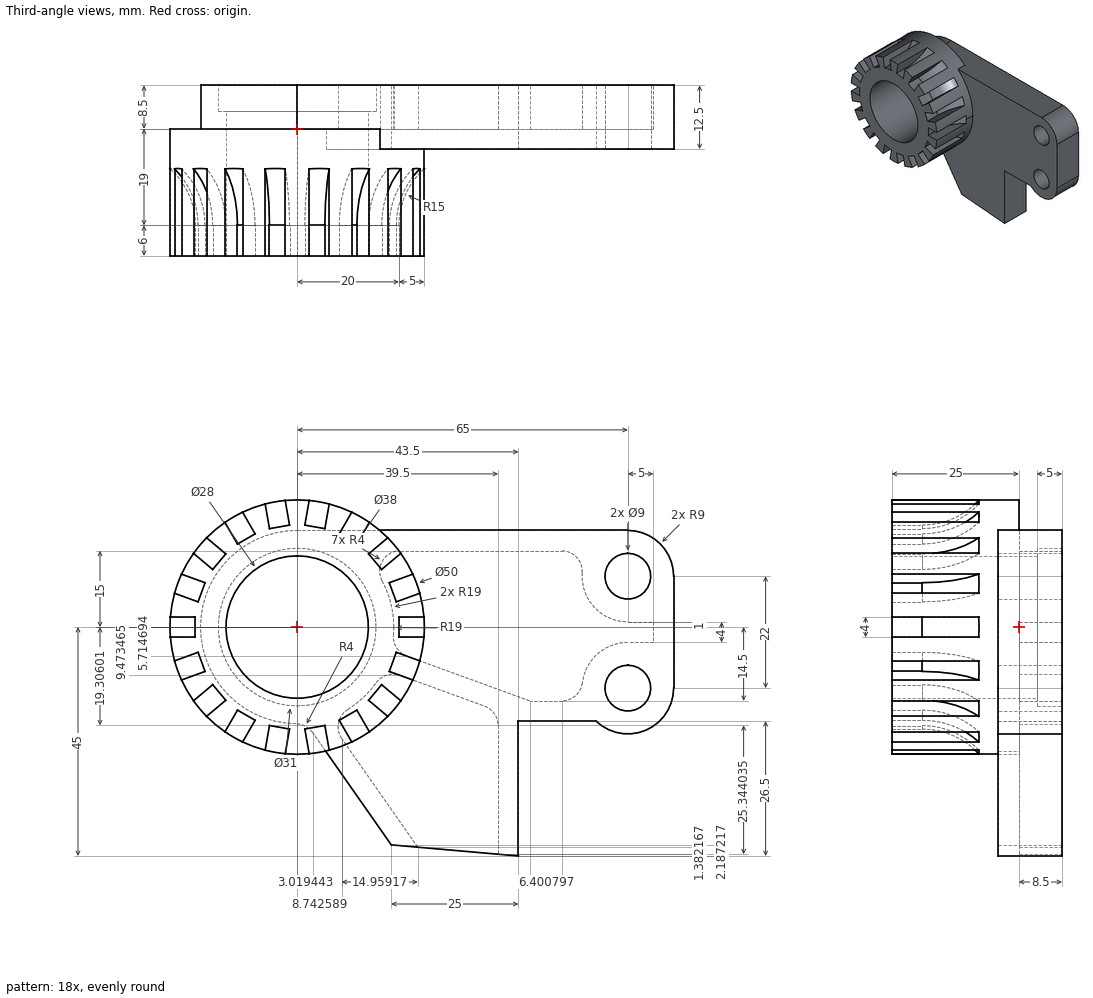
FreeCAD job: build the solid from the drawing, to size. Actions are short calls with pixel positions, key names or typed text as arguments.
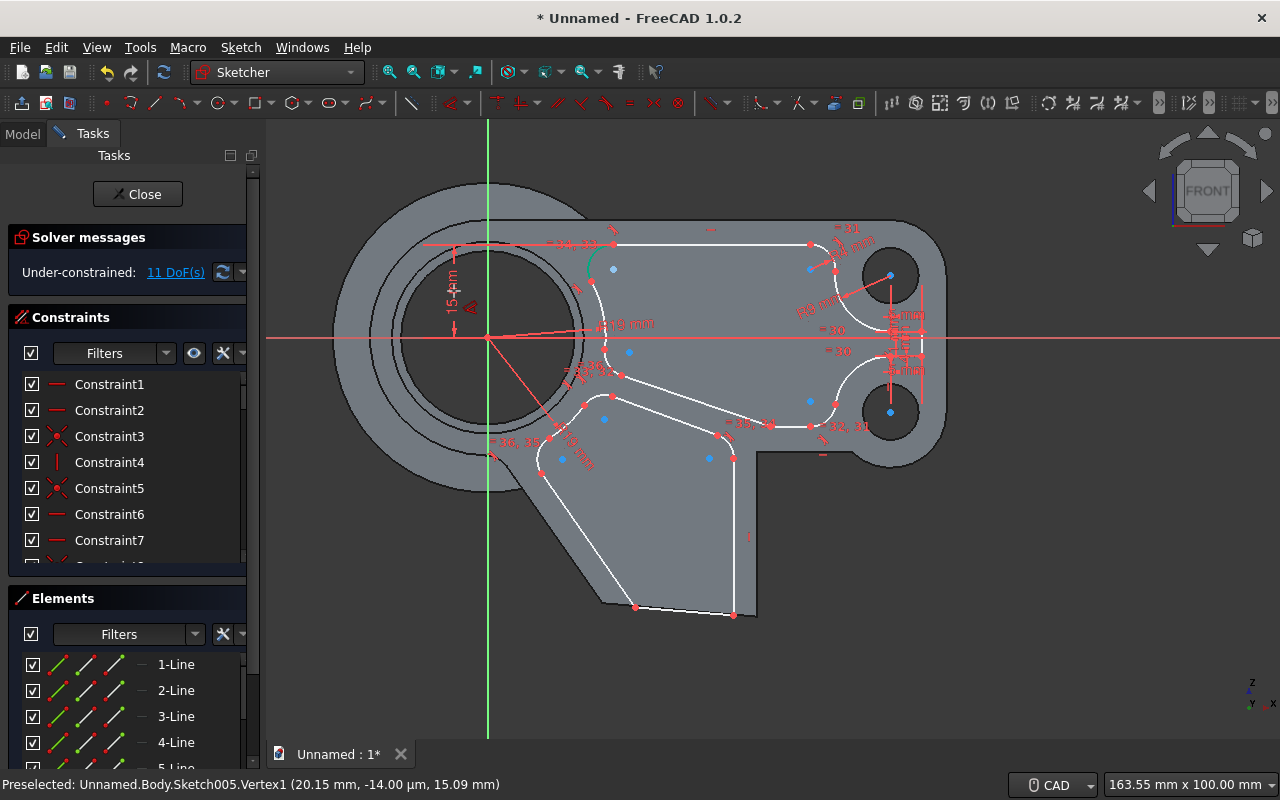
click(891, 332)
click(689, 298)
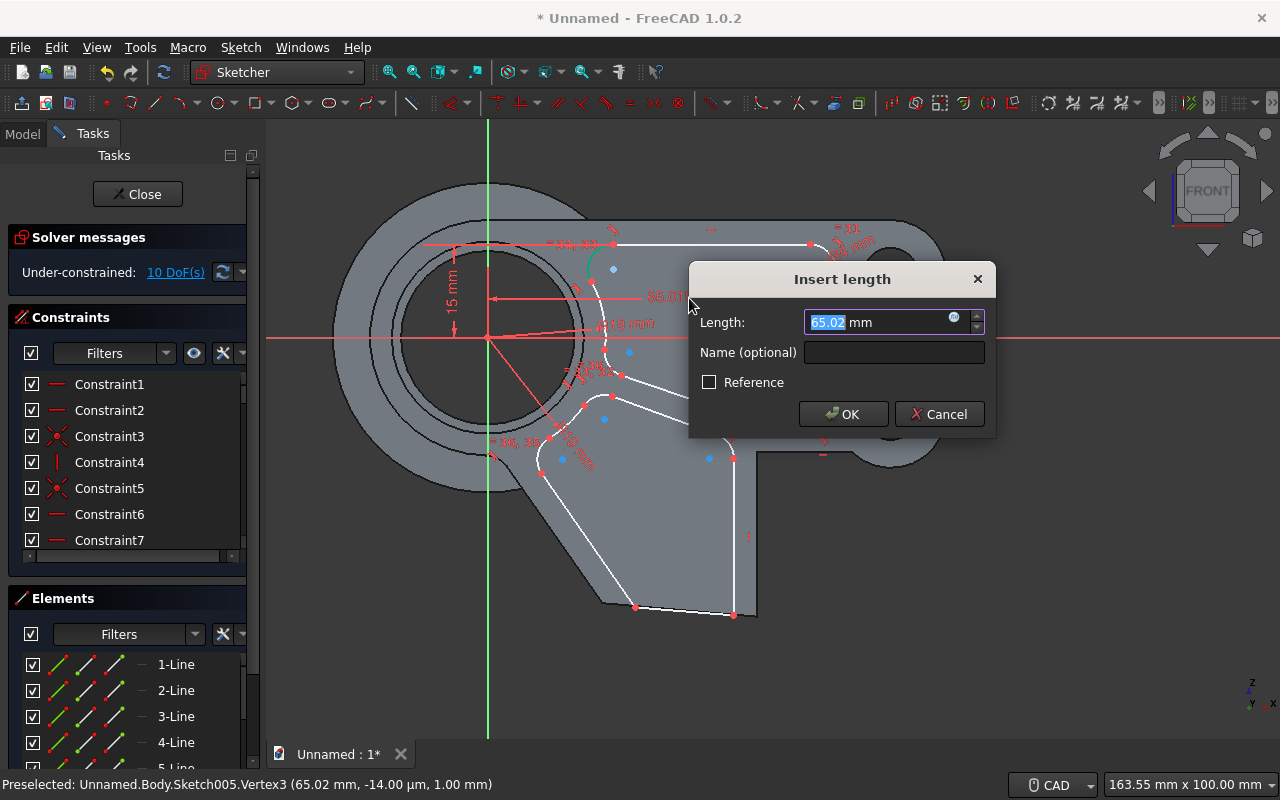
text(65)
key(Return)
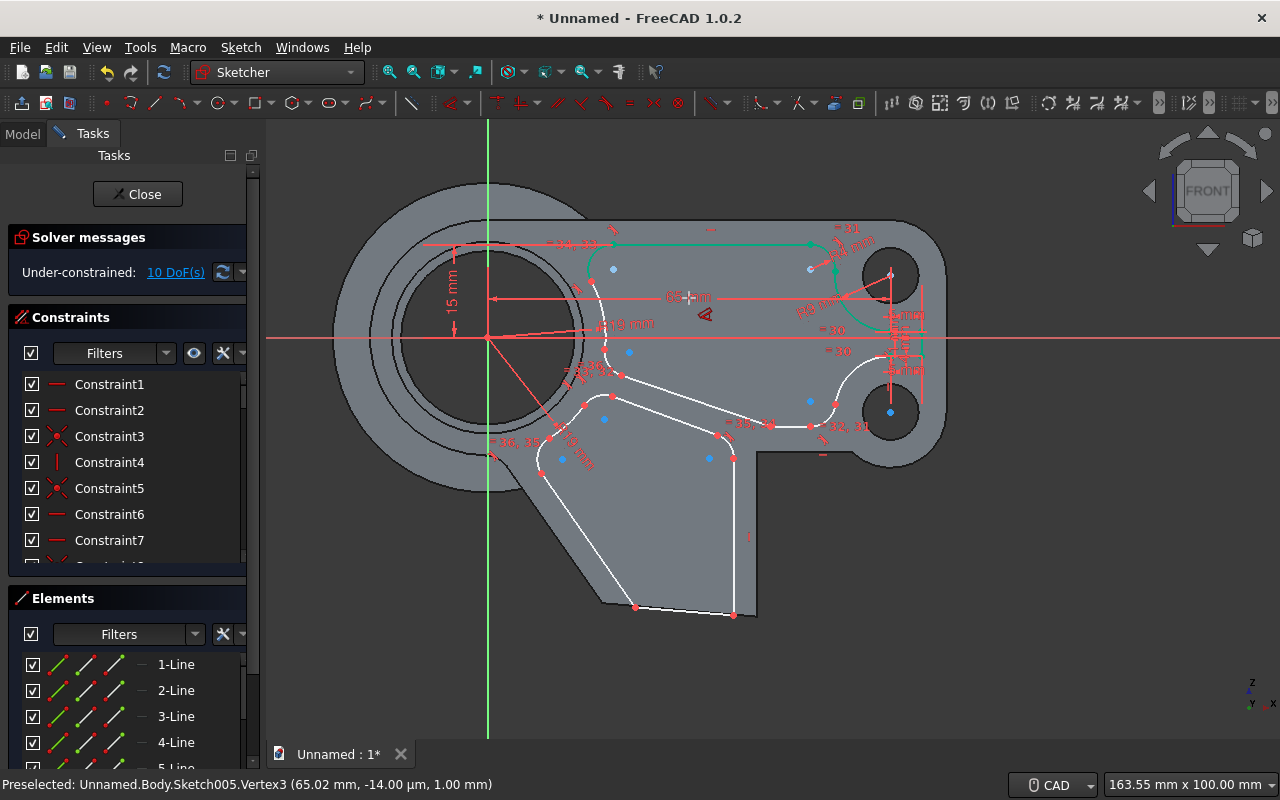
click(811, 427)
click(454, 382)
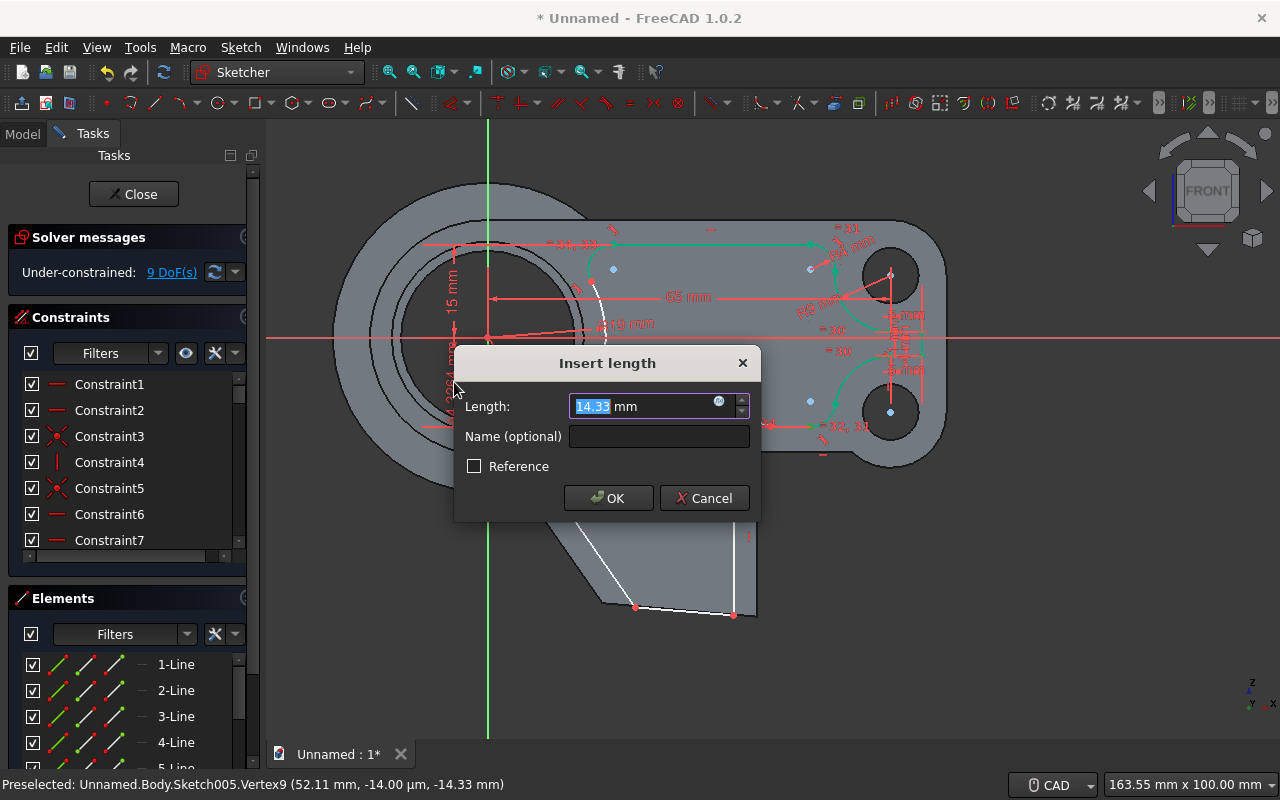
text(14.5)
key(Return)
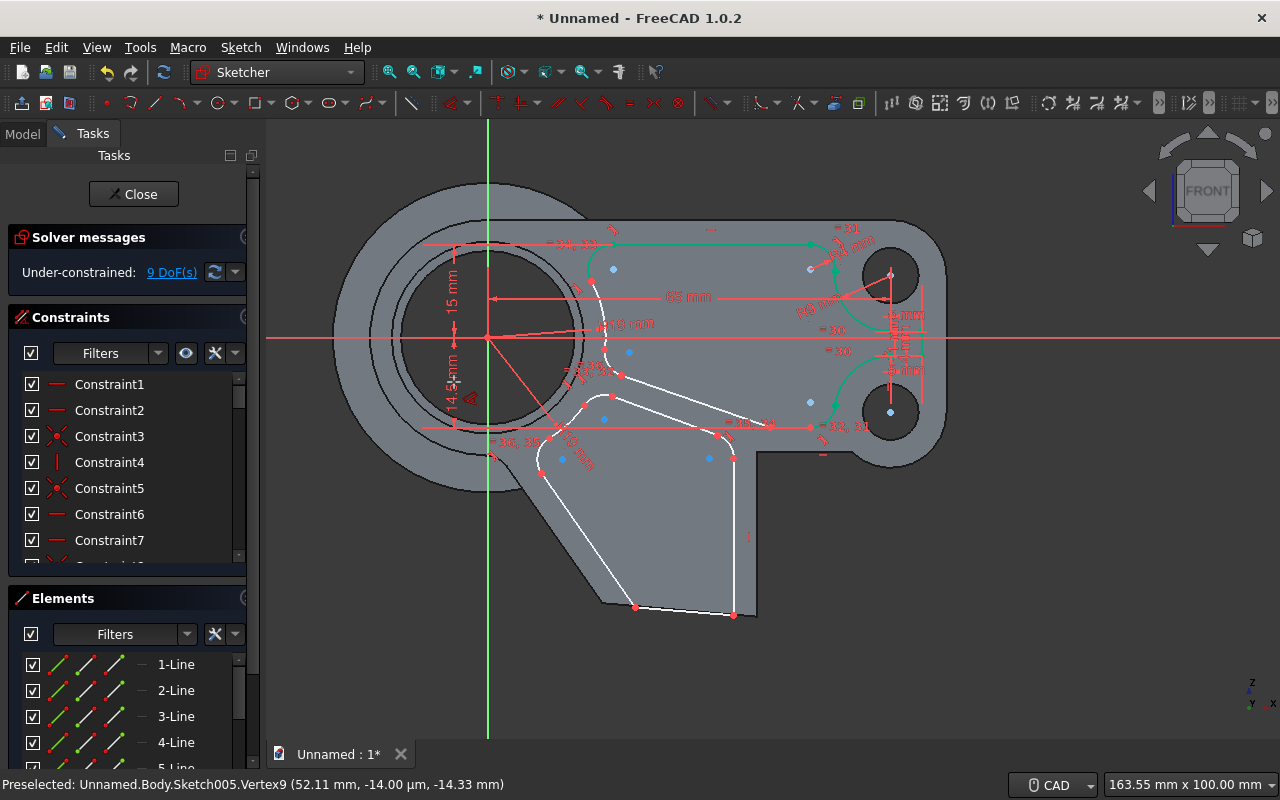
click(734, 458)
click(554, 304)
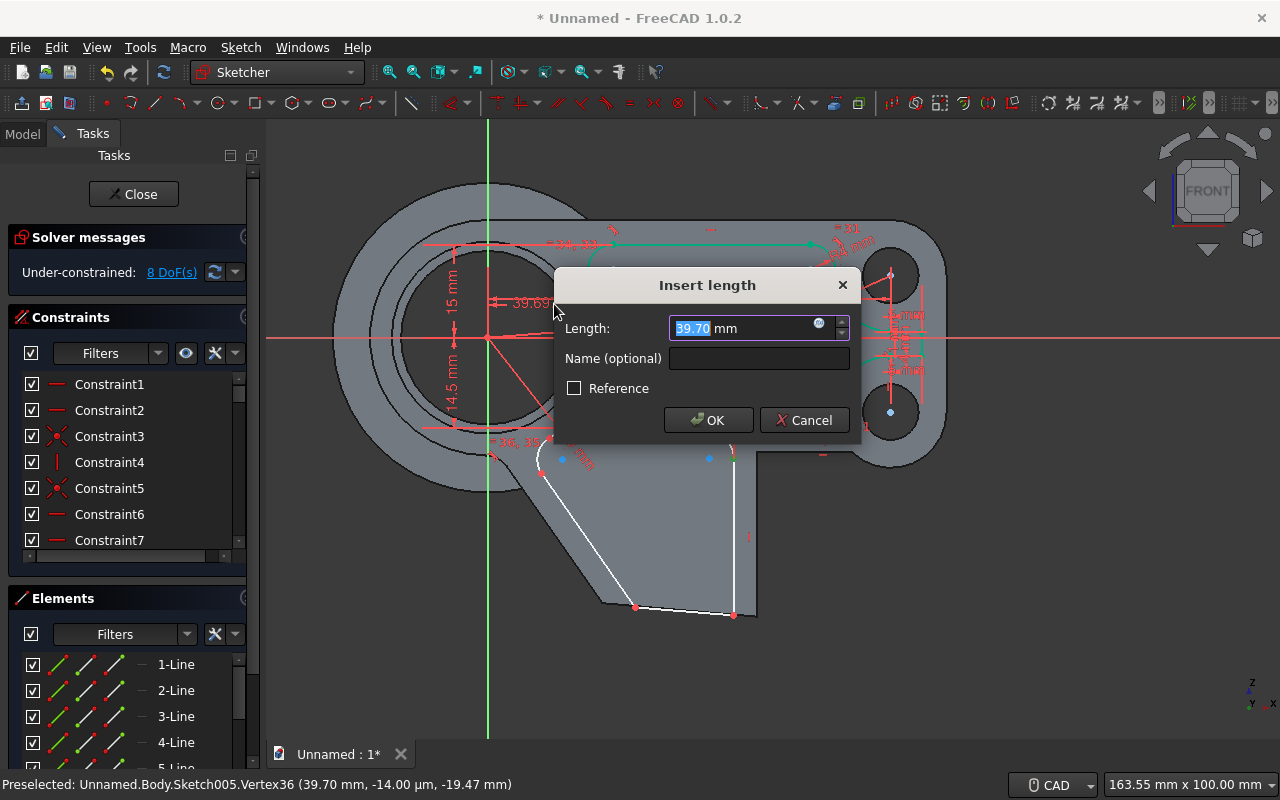
text(39.5)
key(Return)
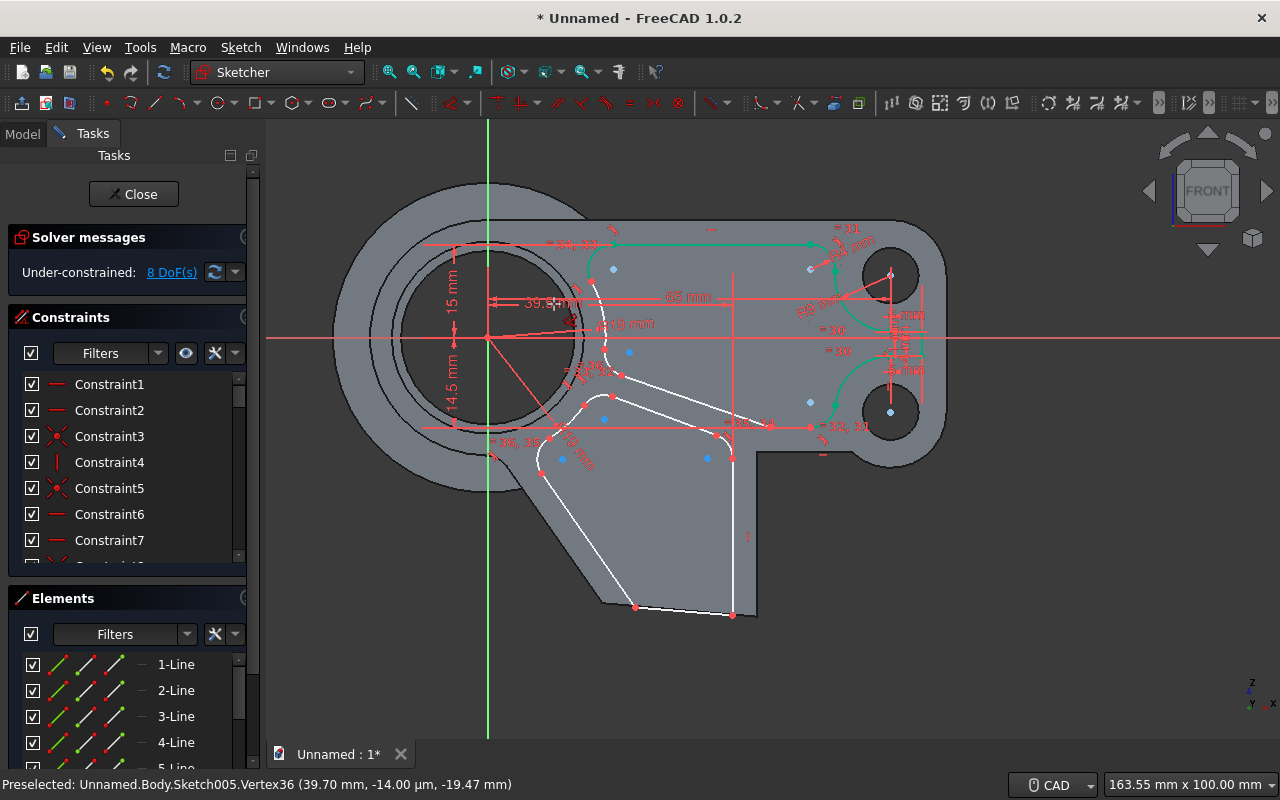
click(799, 428)
click(791, 394)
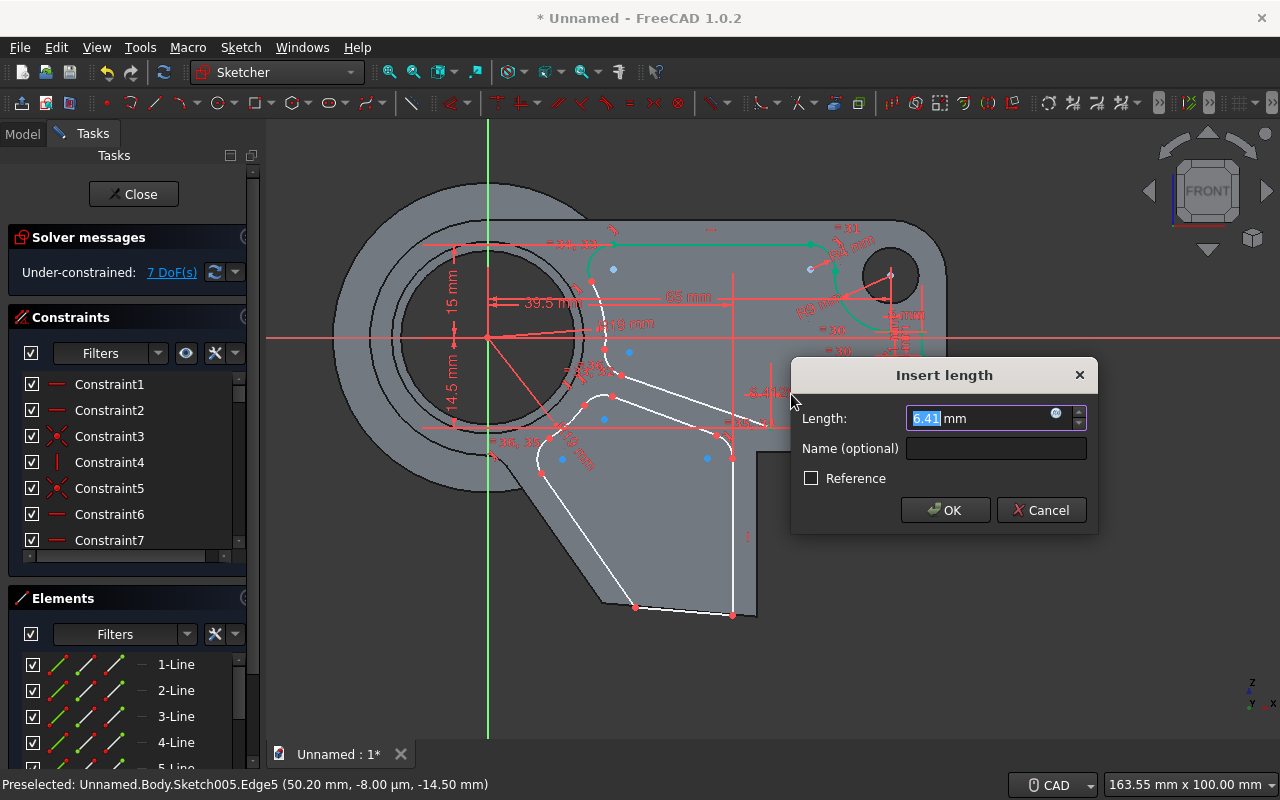
text(6.400797)
key(Return)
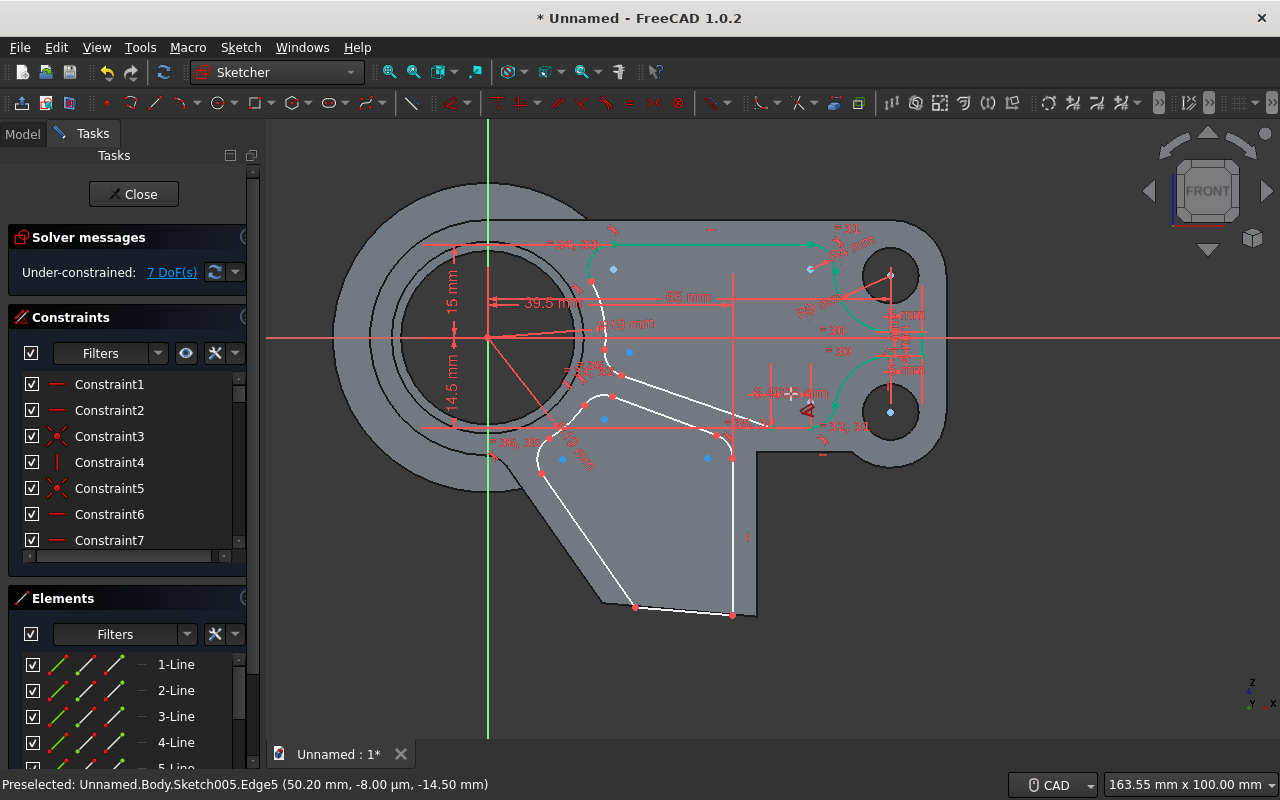
click(733, 506)
click(767, 537)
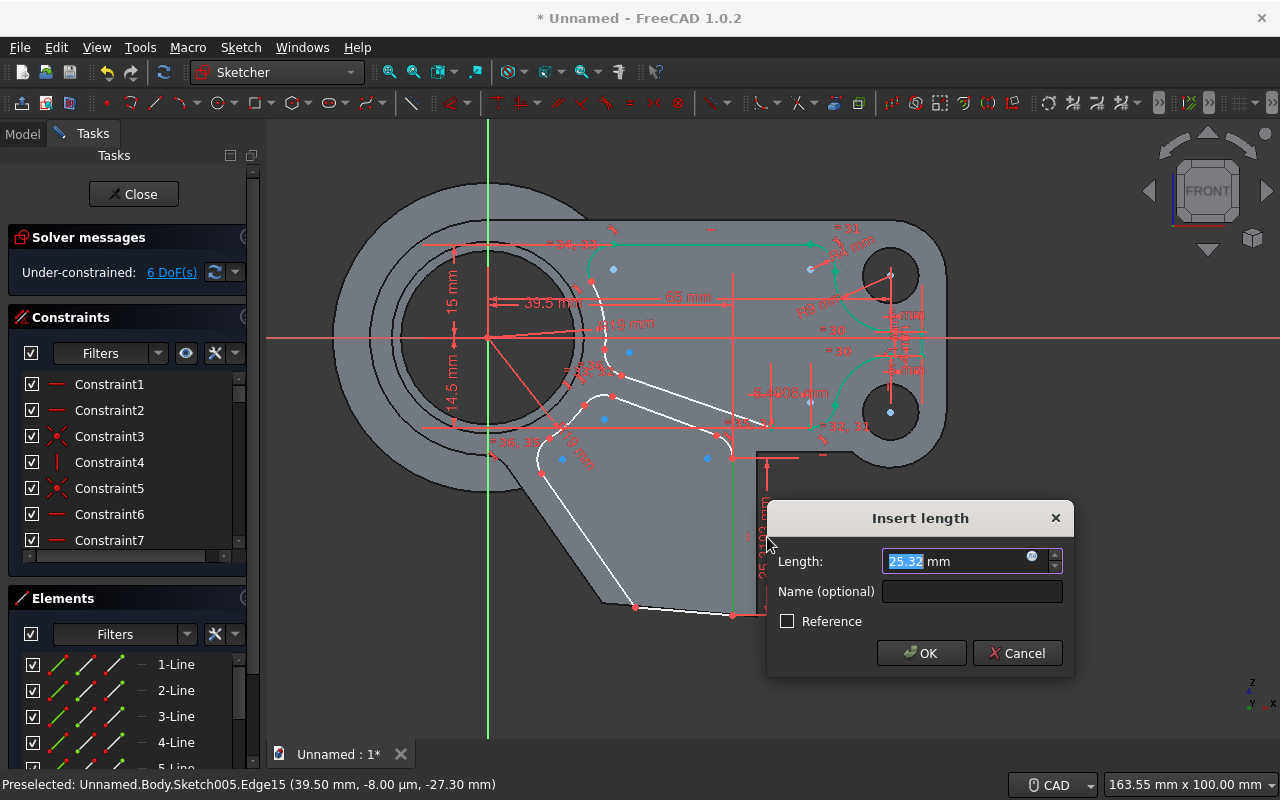
text(25.344035)
key(Return)